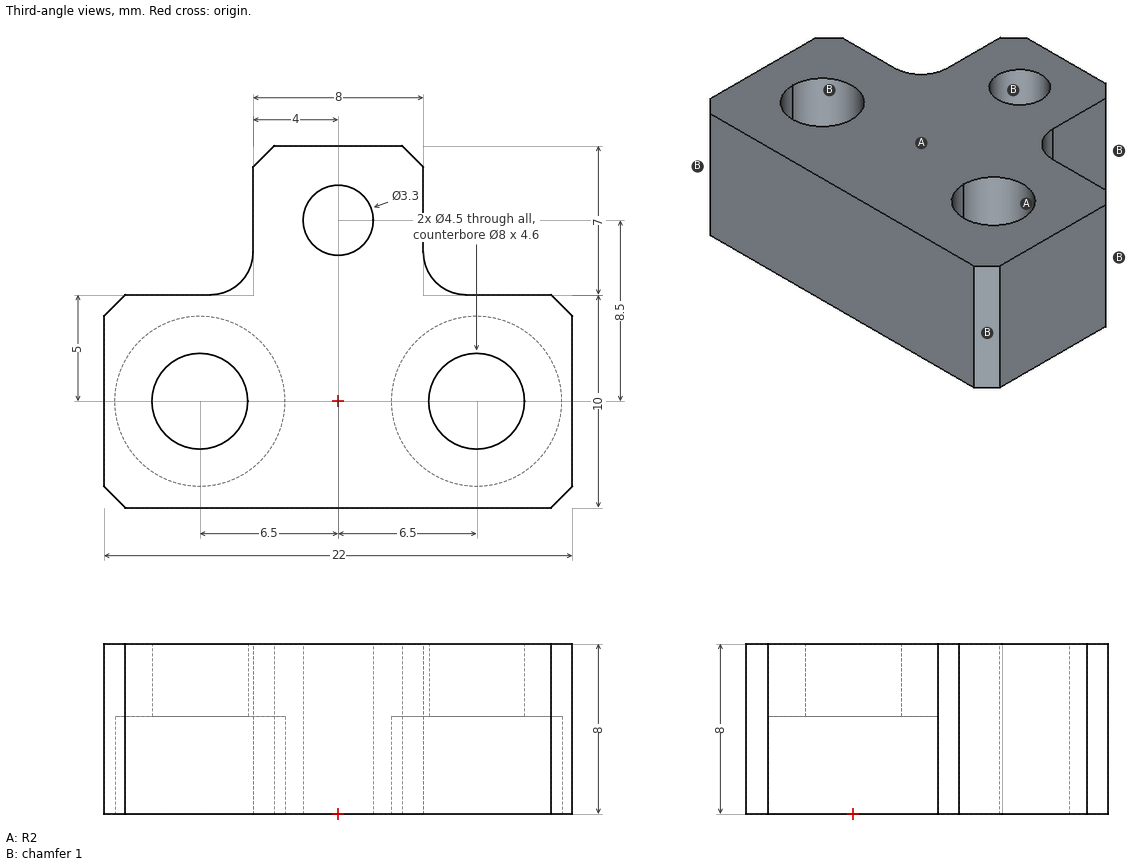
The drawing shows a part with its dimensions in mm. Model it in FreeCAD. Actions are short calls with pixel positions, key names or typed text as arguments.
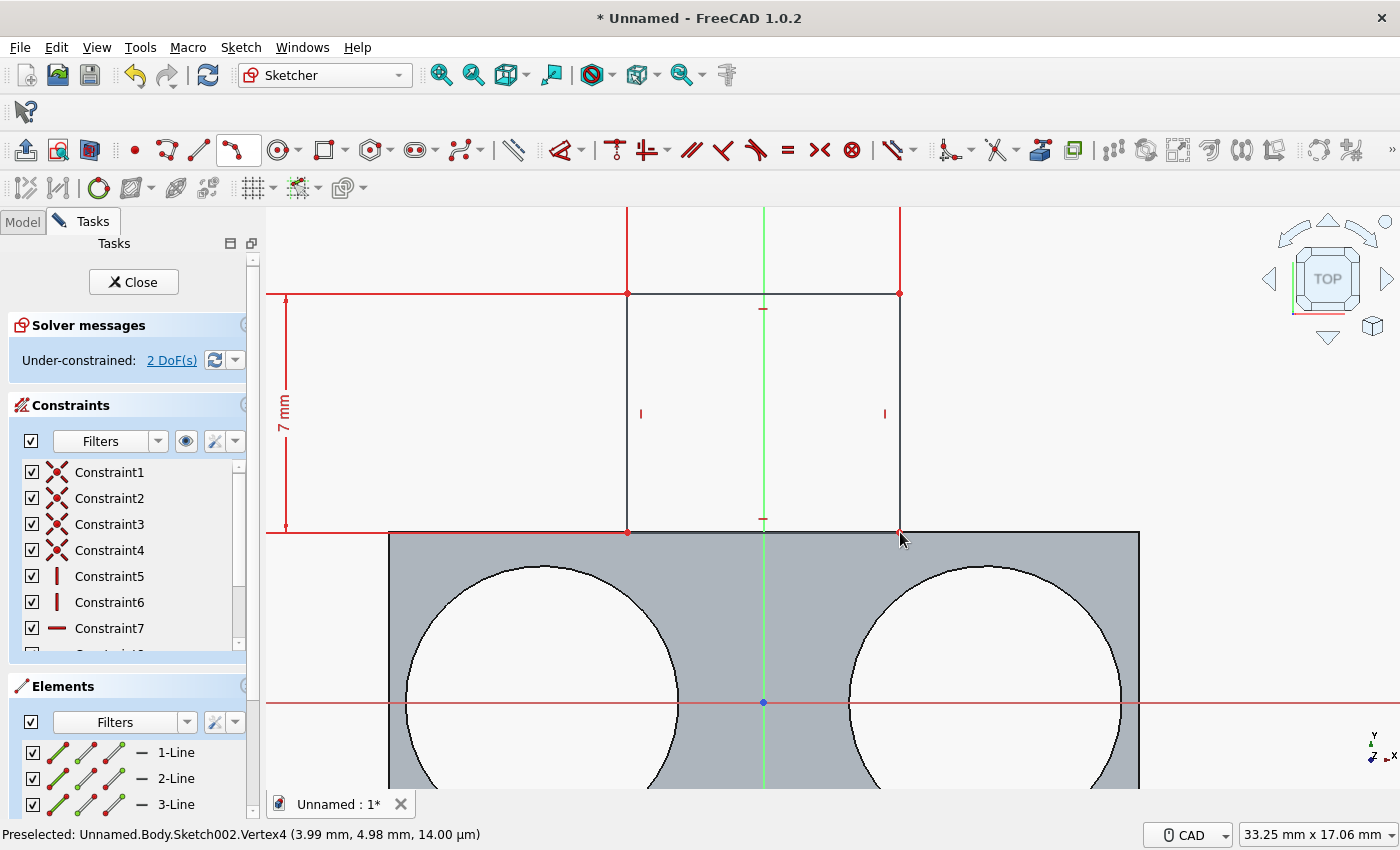
click(560, 150)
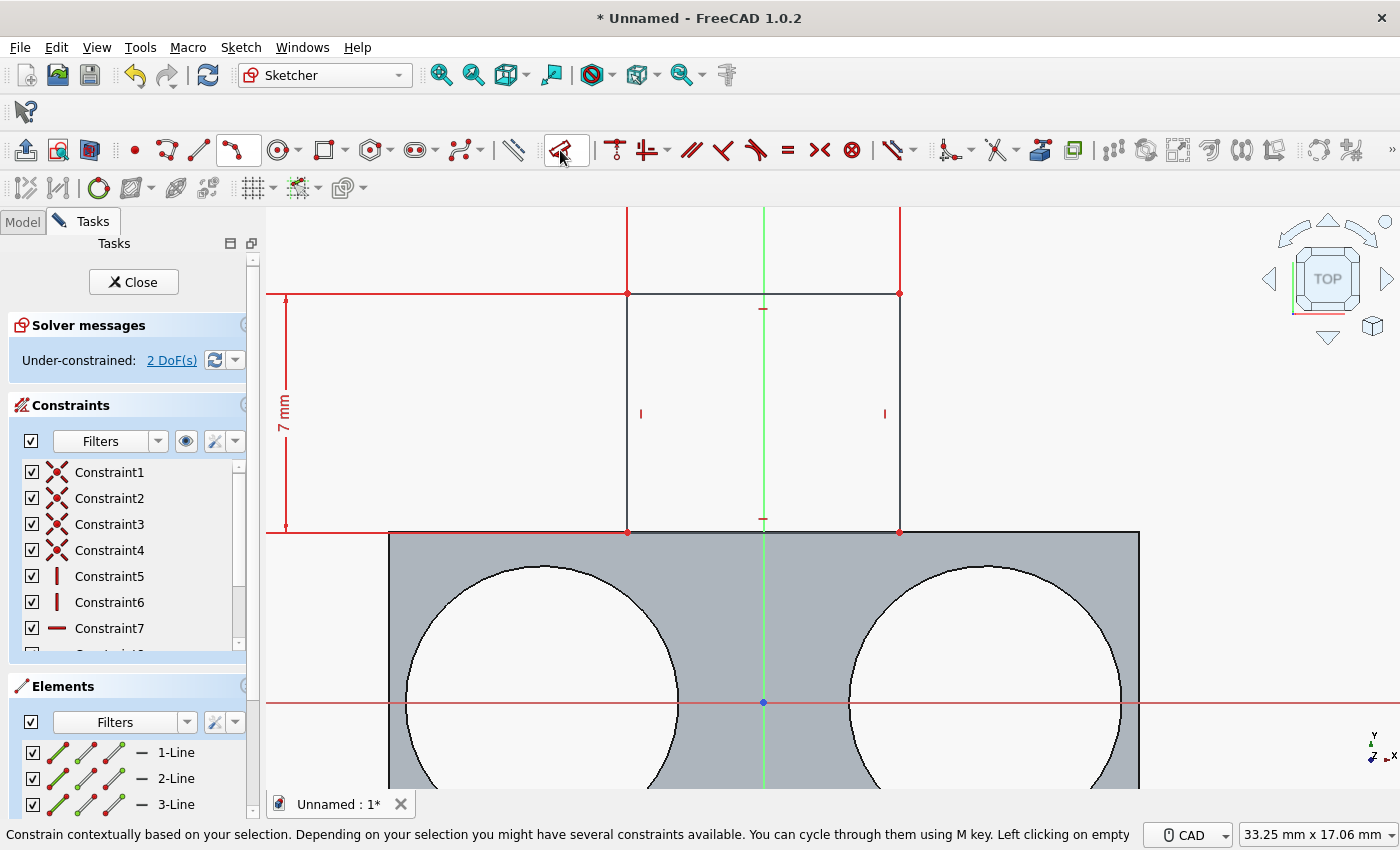
click(627, 294)
click(695, 737)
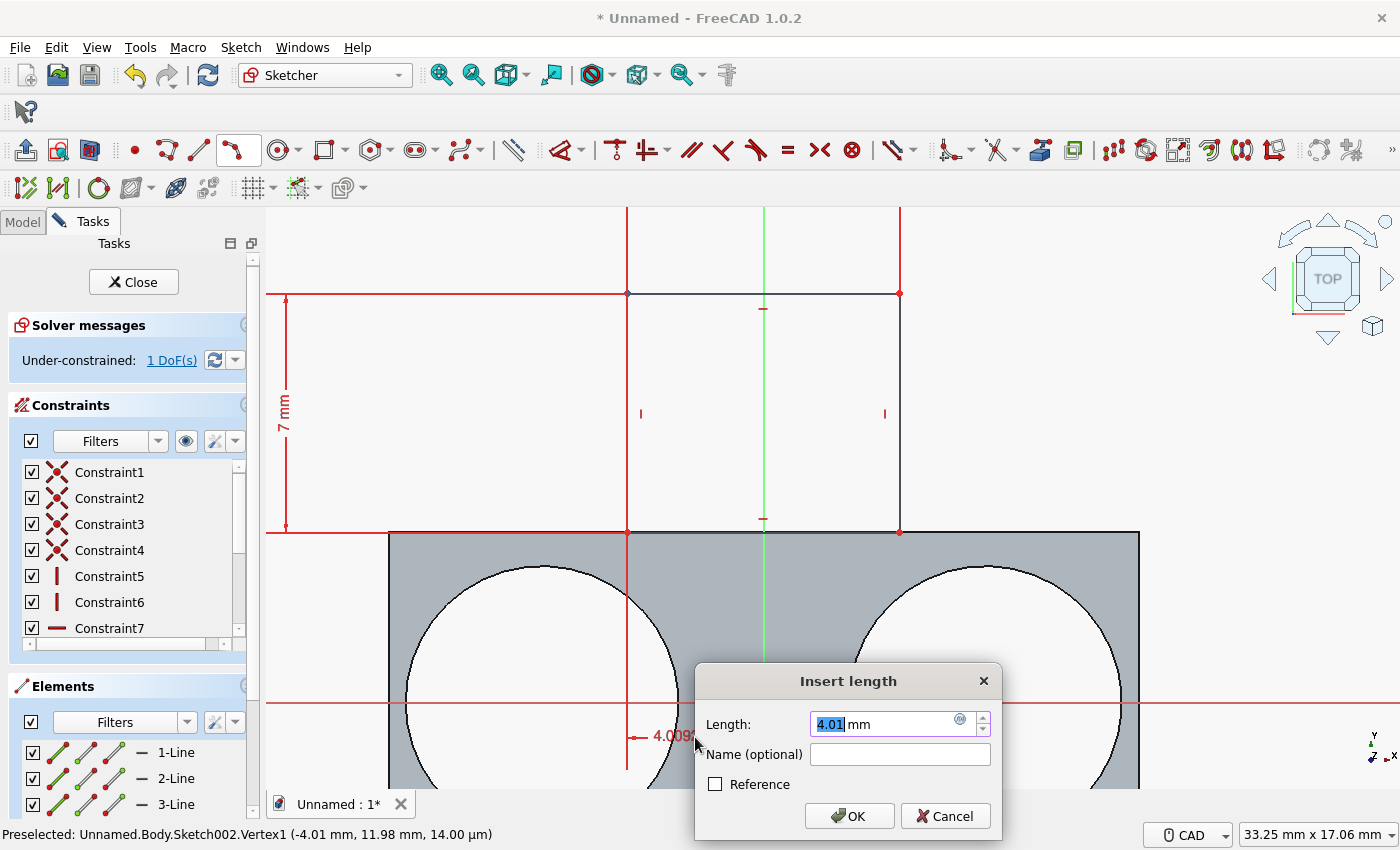
text(4)
key(Return)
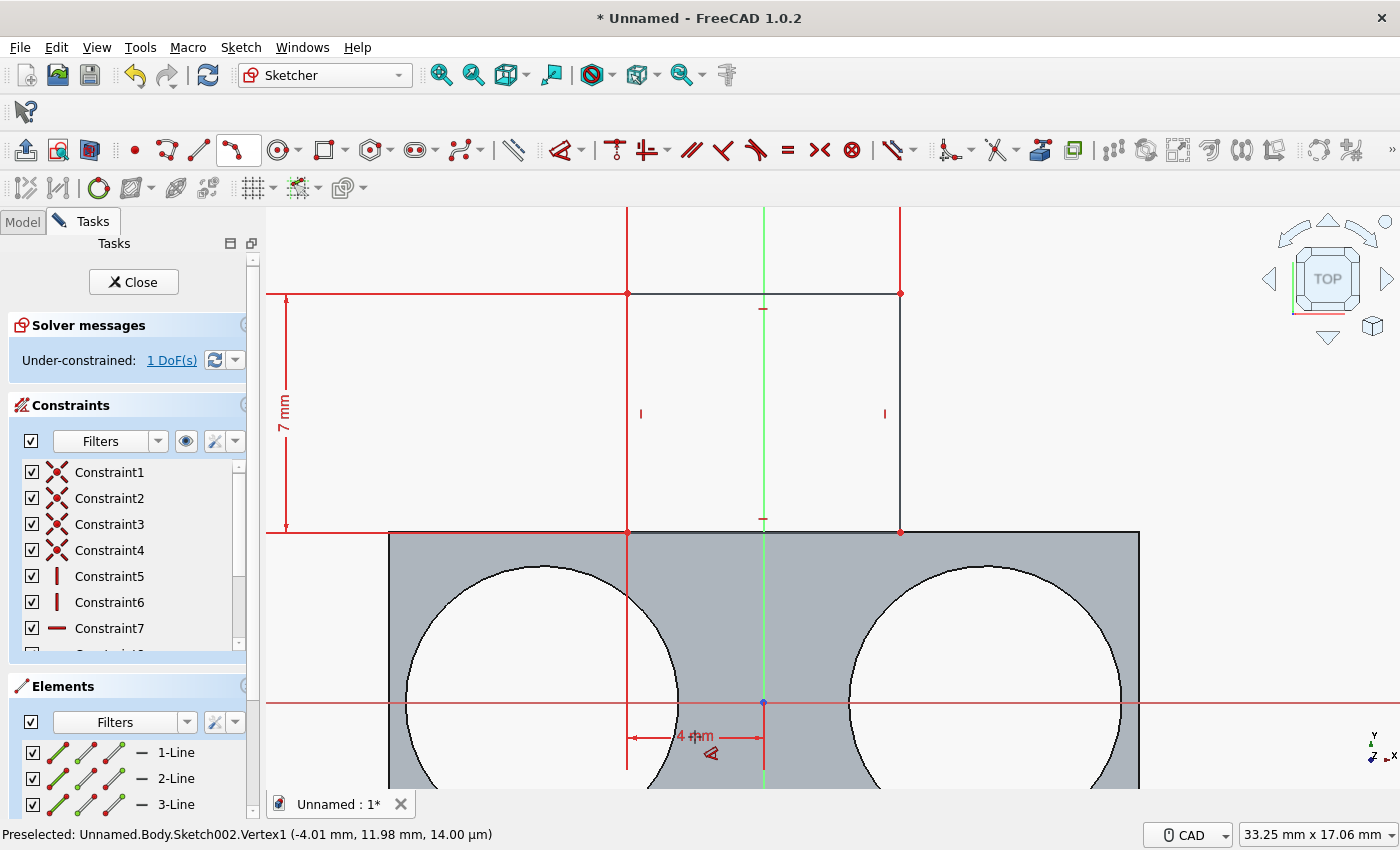
click(627, 533)
click(593, 618)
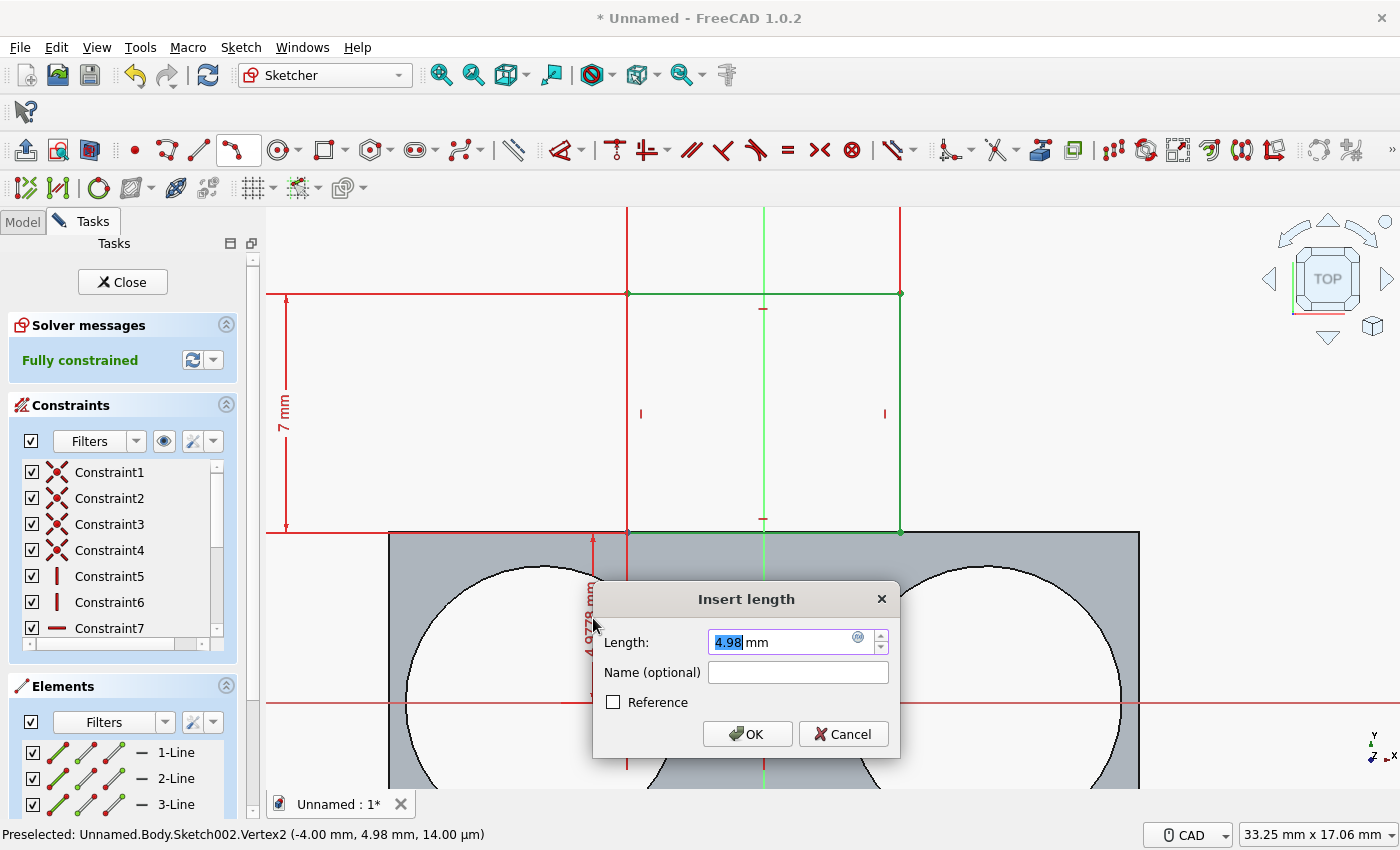
text(5)
key(Return)
key(Escape)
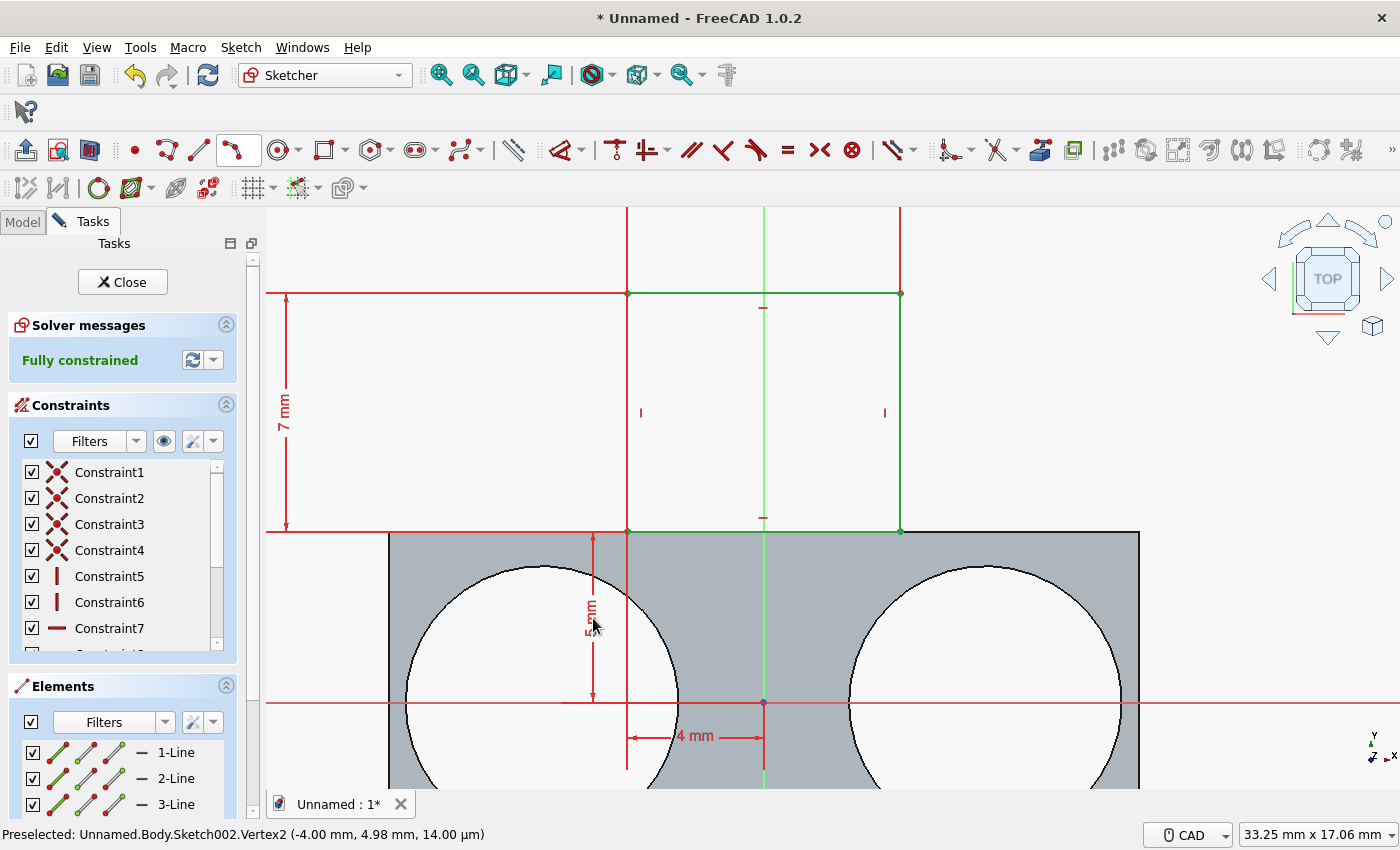
click(123, 282)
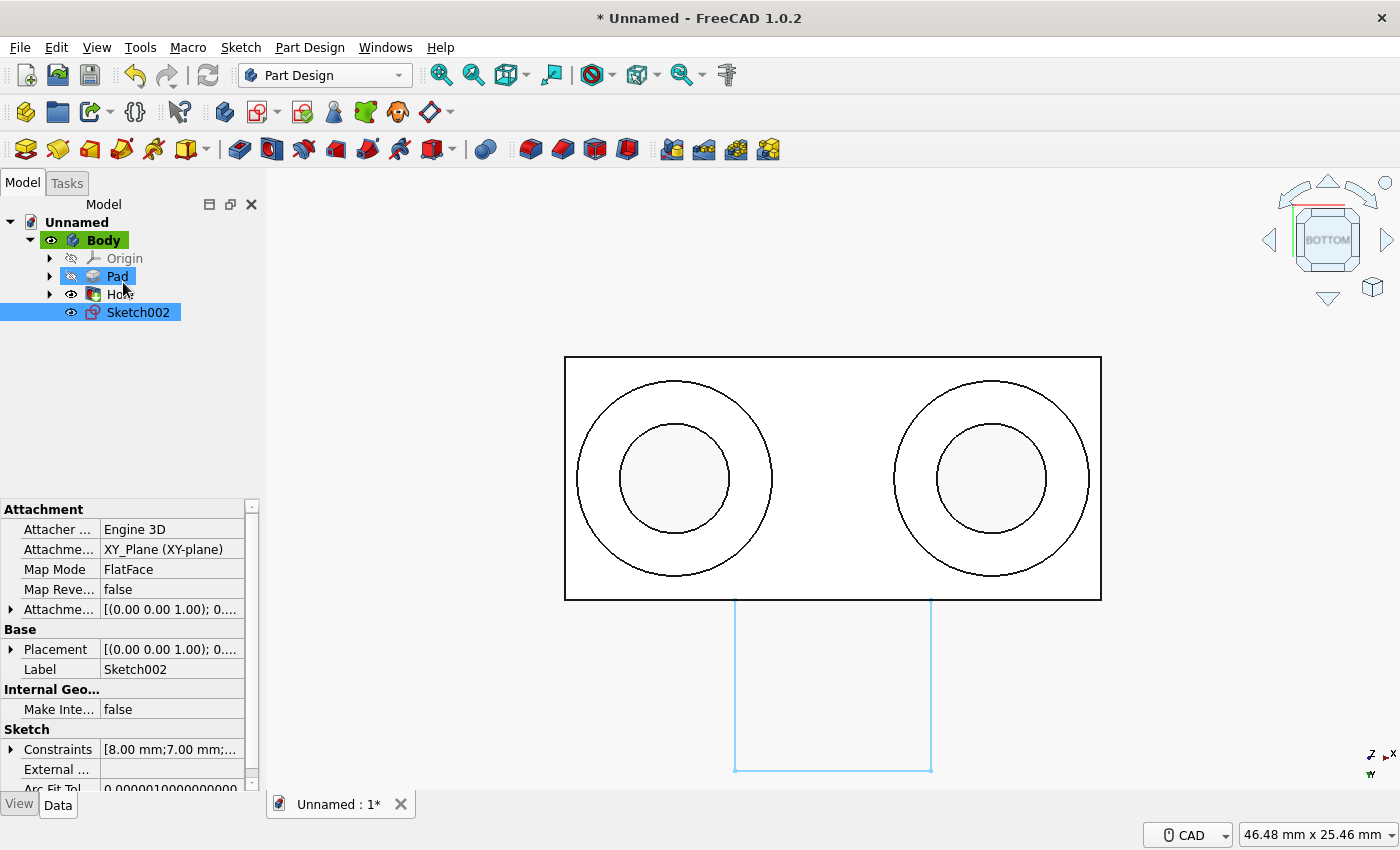
click(26, 150)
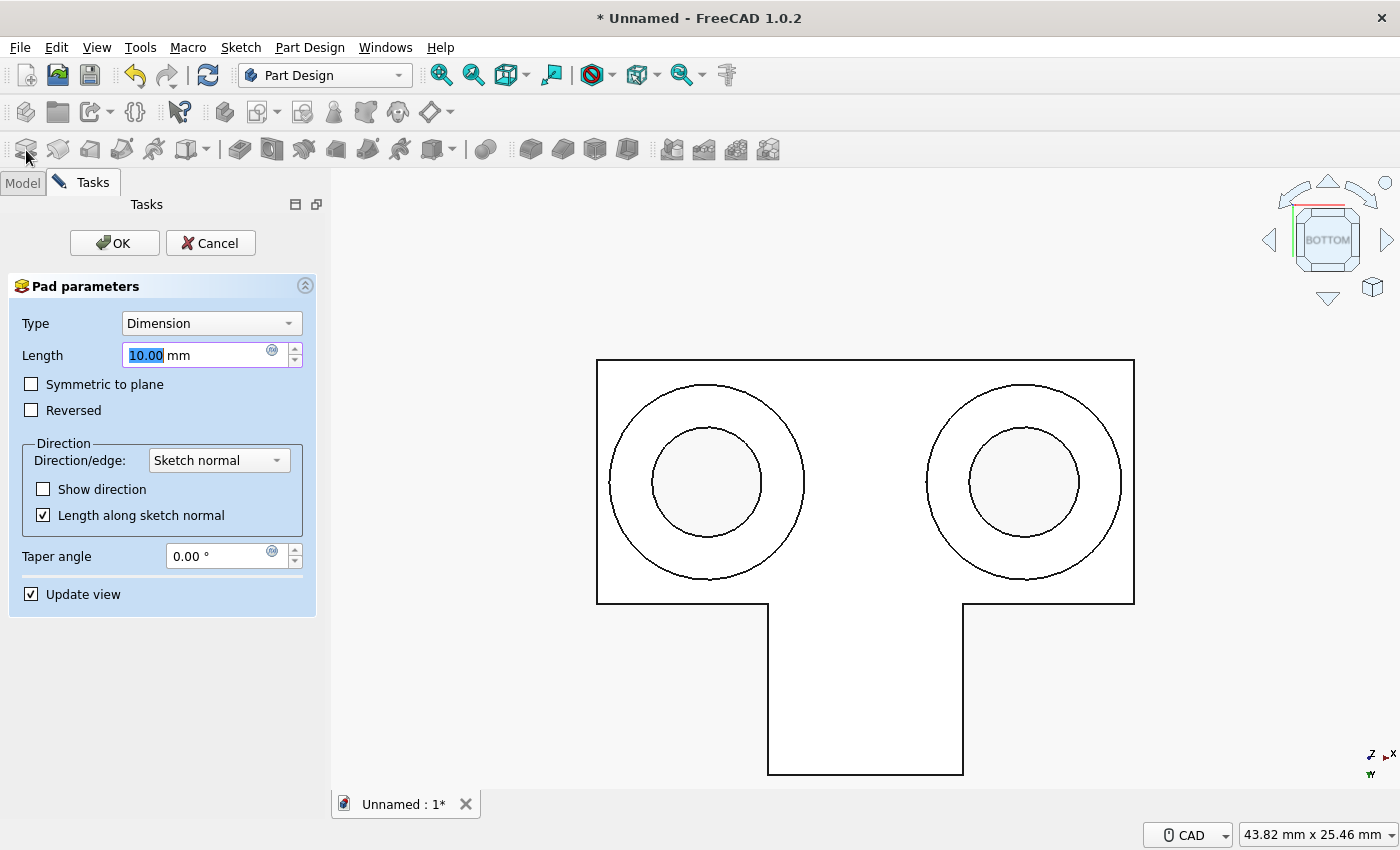
text(8)
key(Tab)